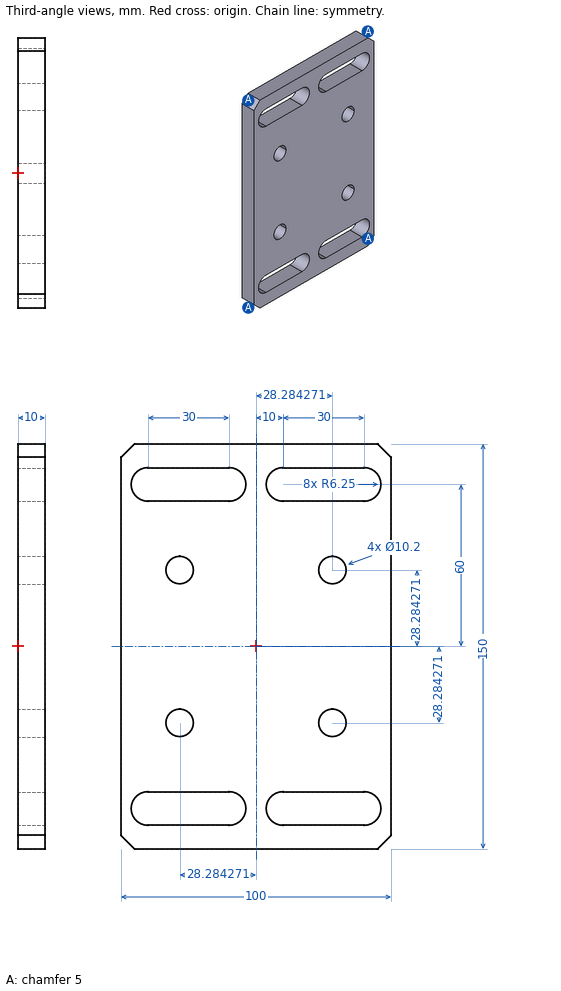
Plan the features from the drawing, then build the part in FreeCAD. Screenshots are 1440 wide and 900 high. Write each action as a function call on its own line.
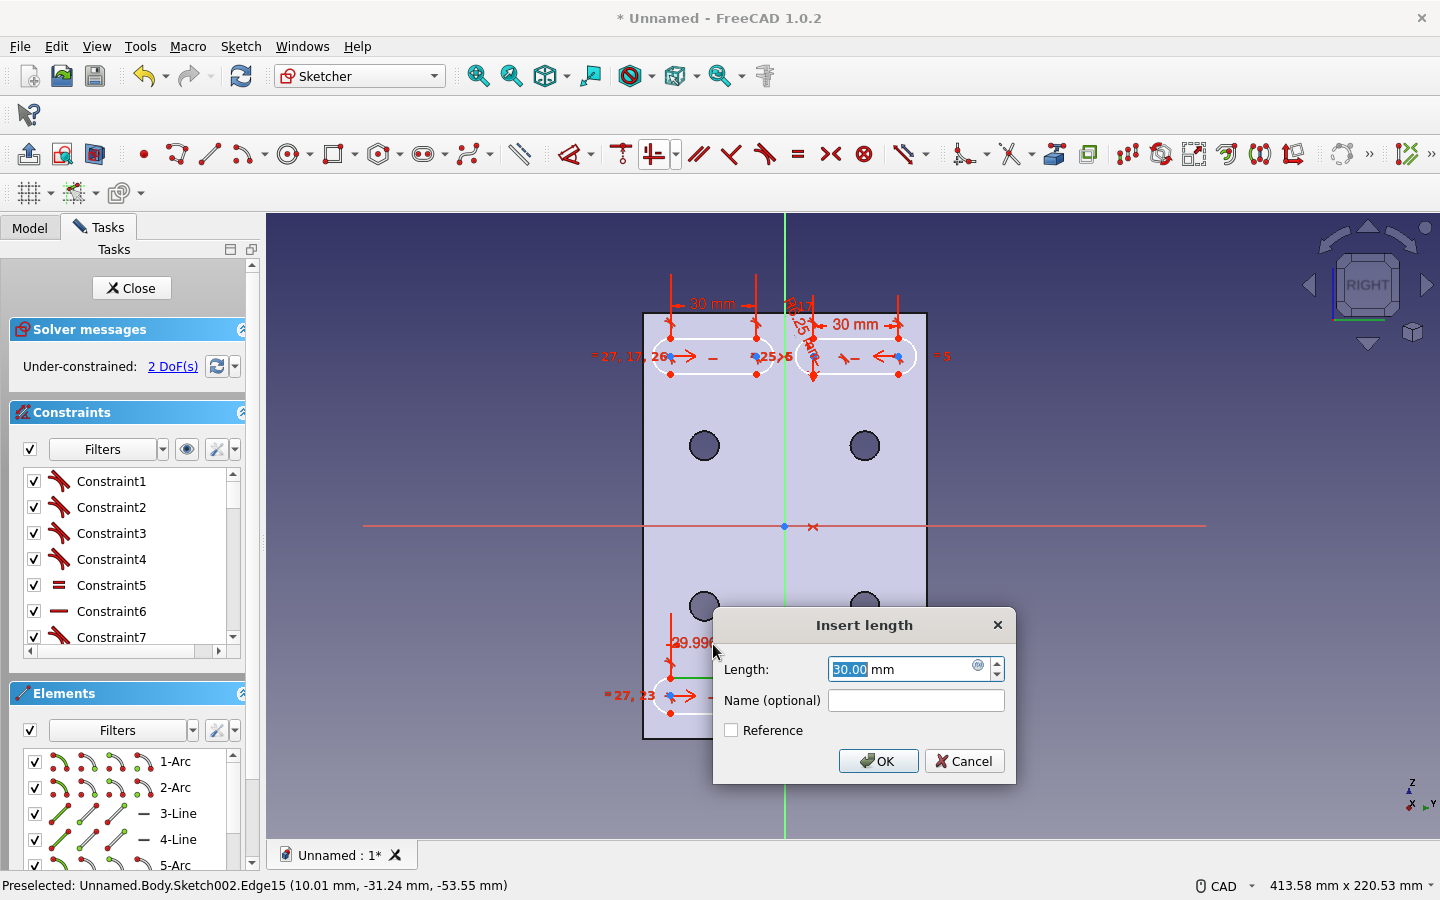
text(30)
key(Return)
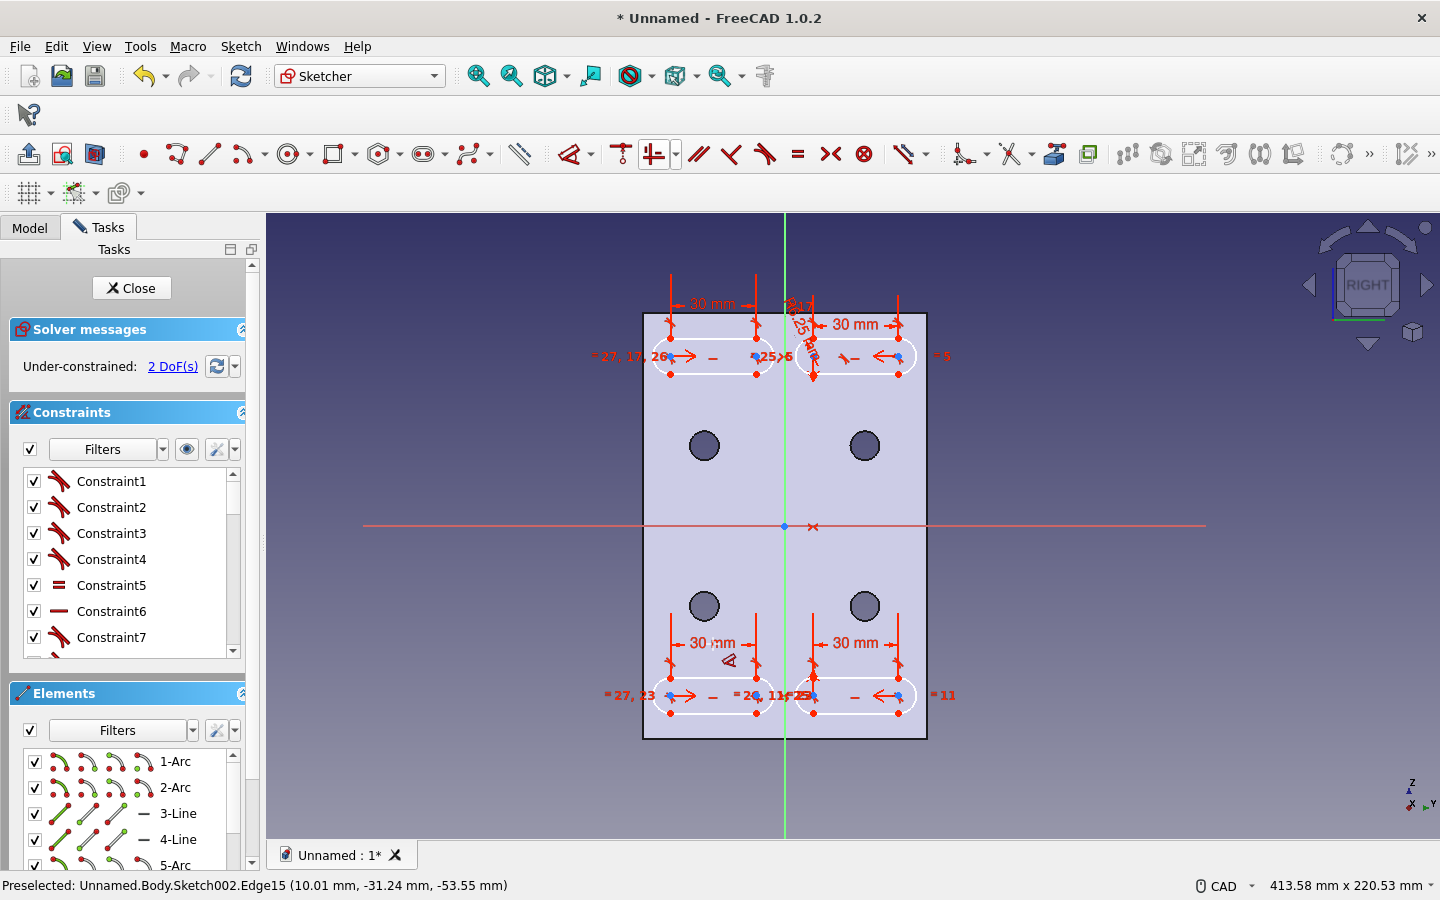
scroll(813, 339, up, 2)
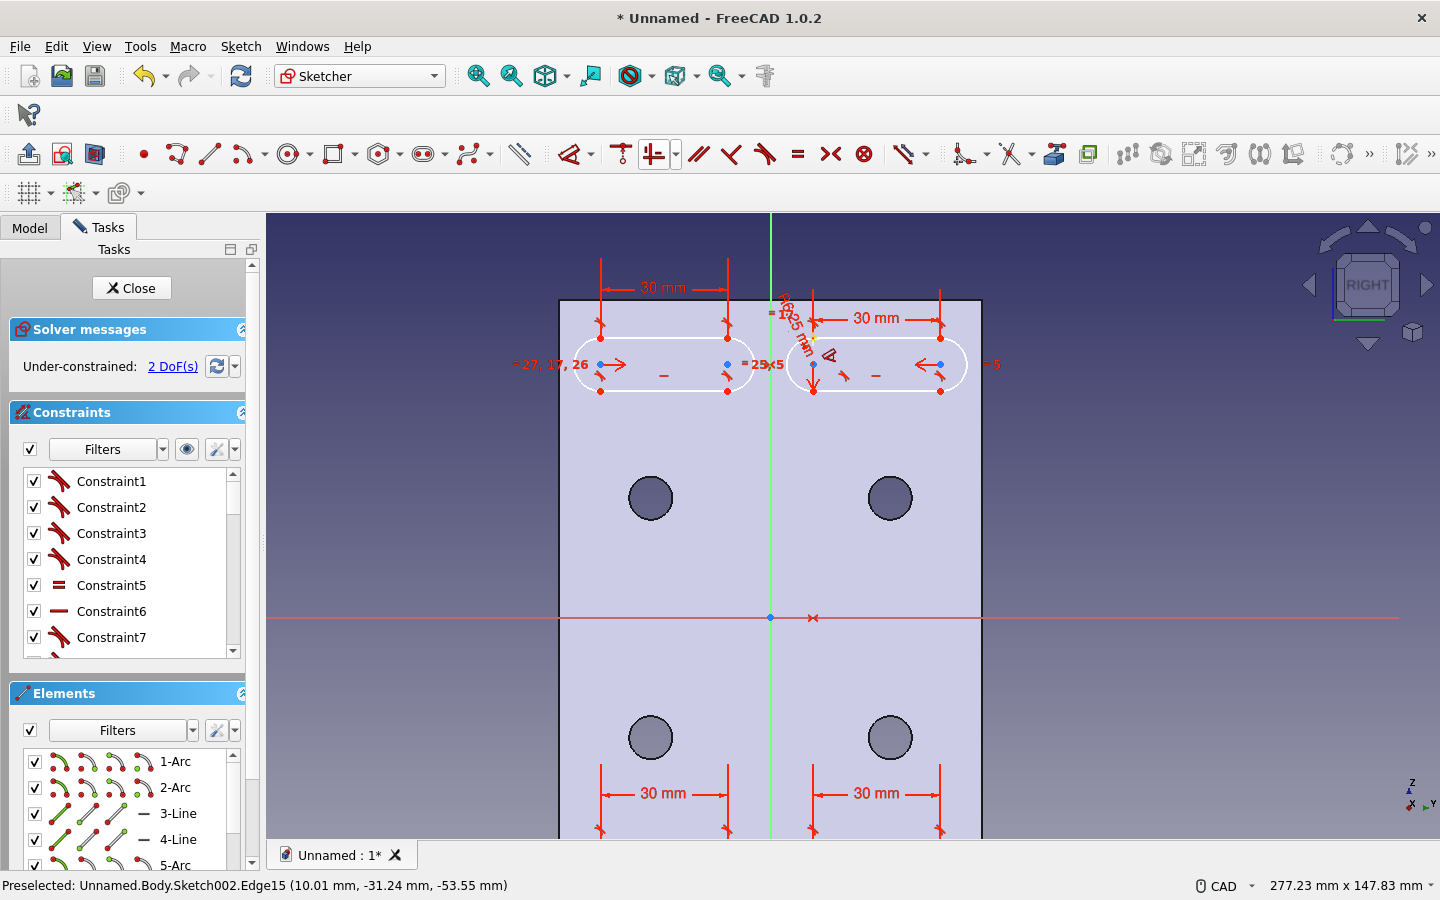
click(813, 338)
click(792, 304)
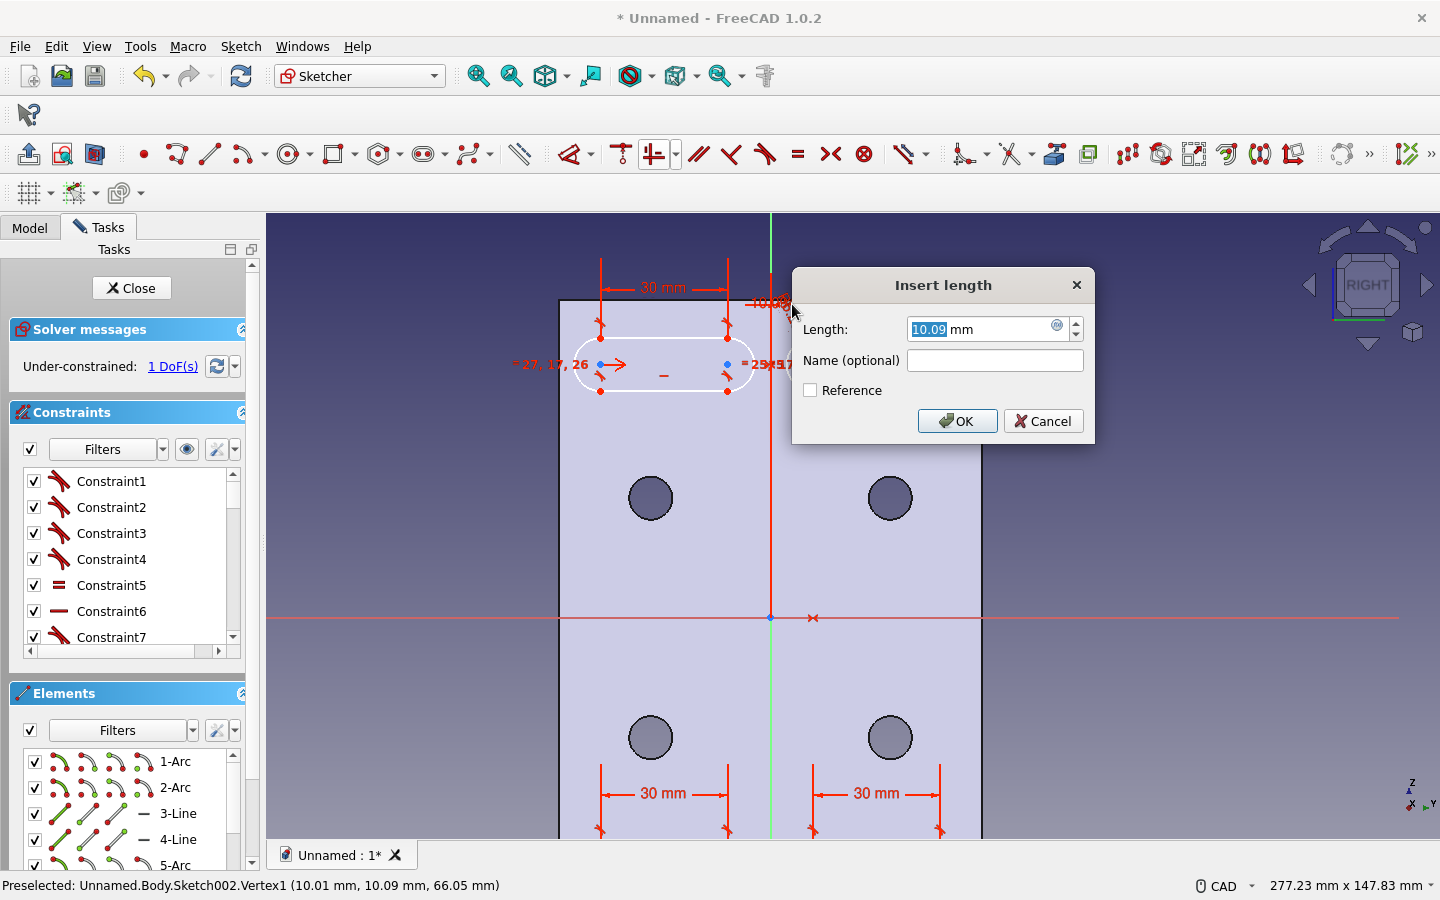
text(10)
key(Return)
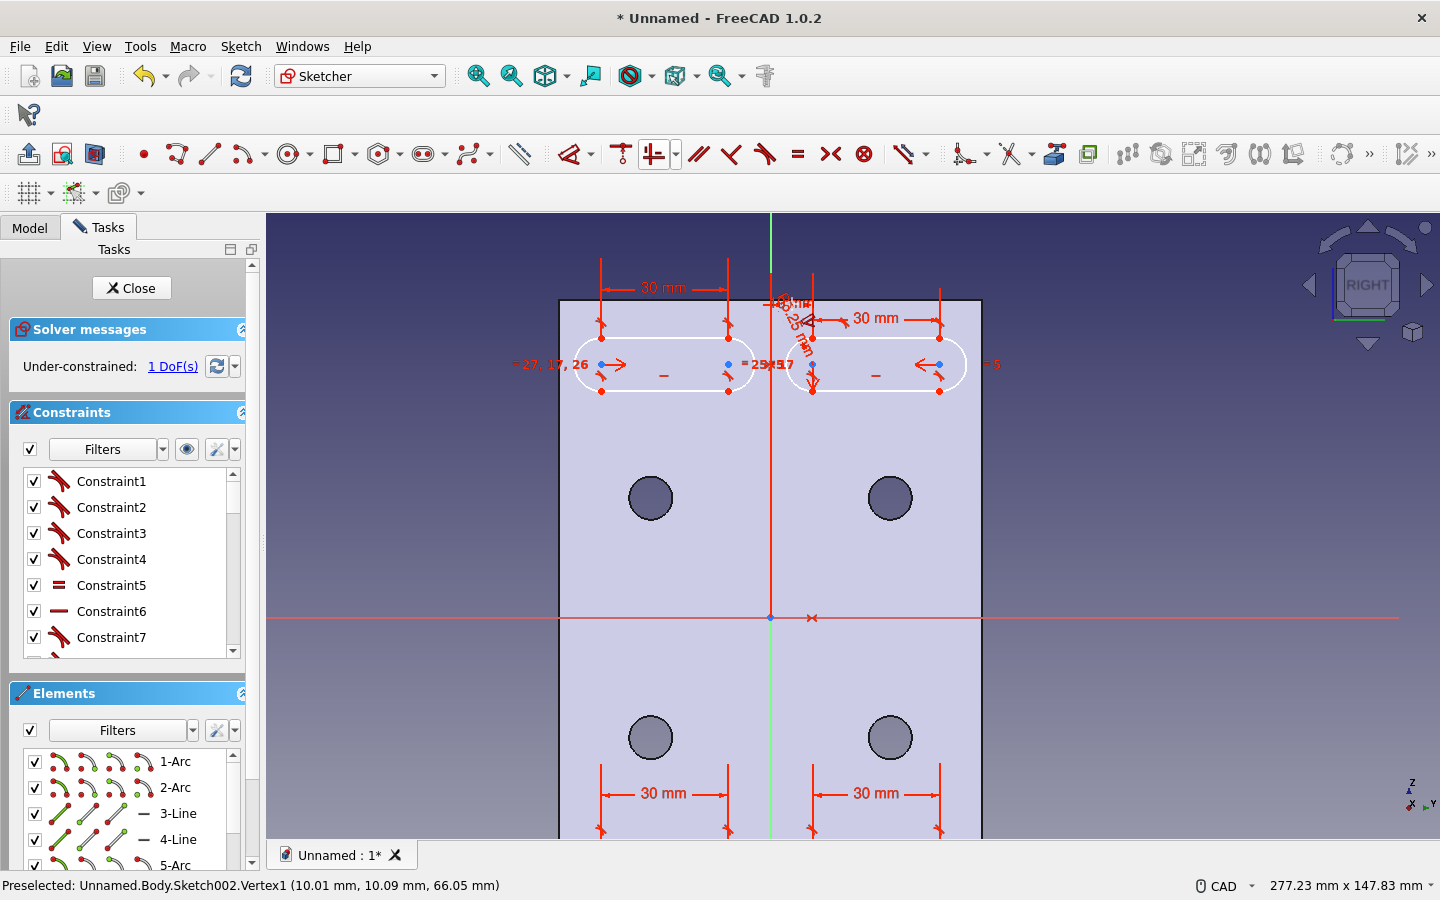
click(813, 365)
click(847, 491)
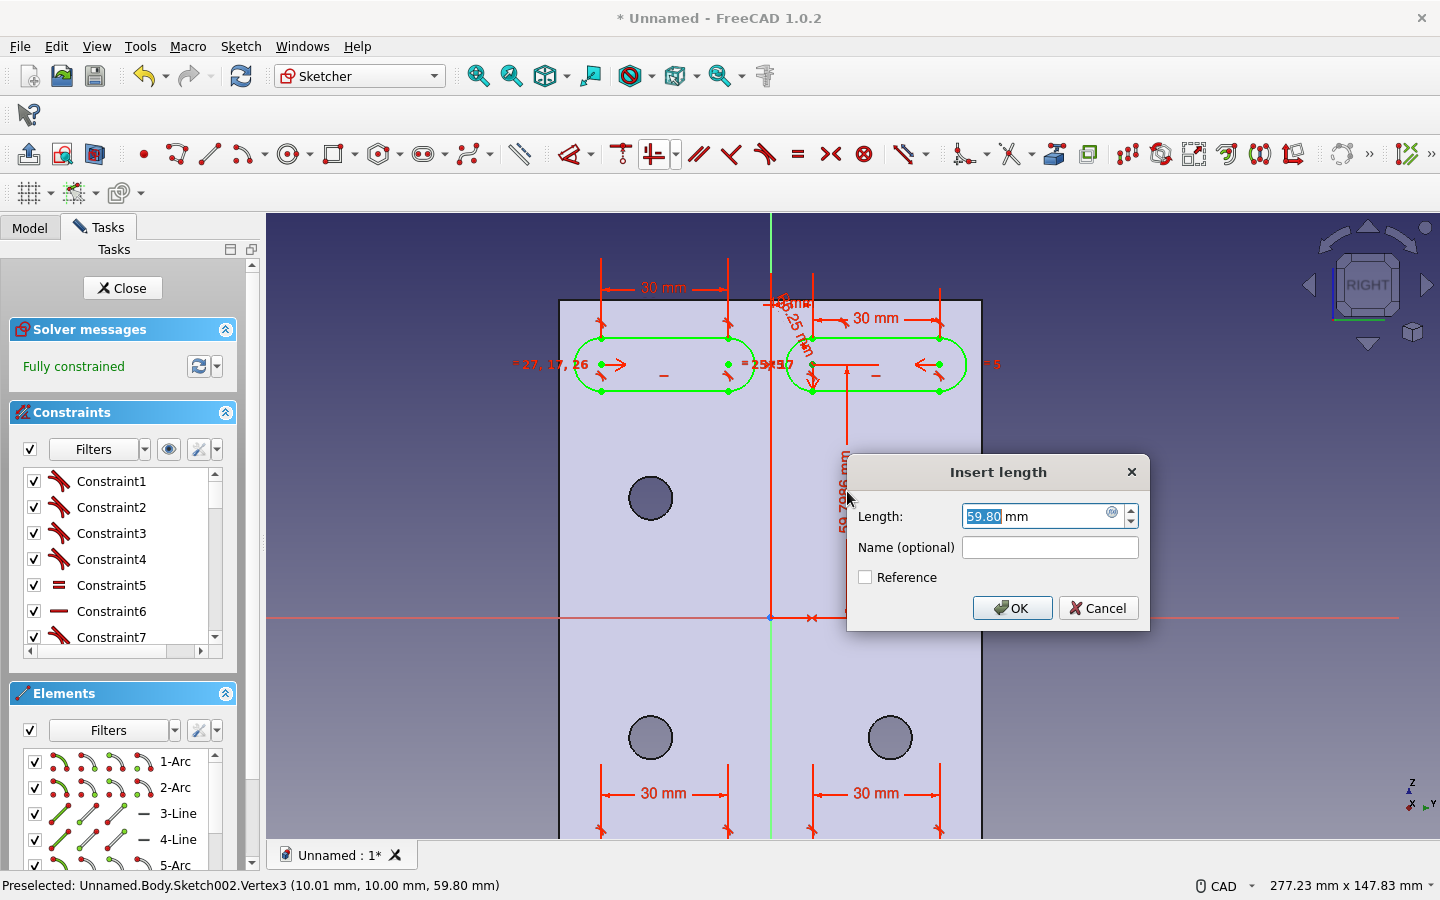
text(60)
key(Return)
key(Escape)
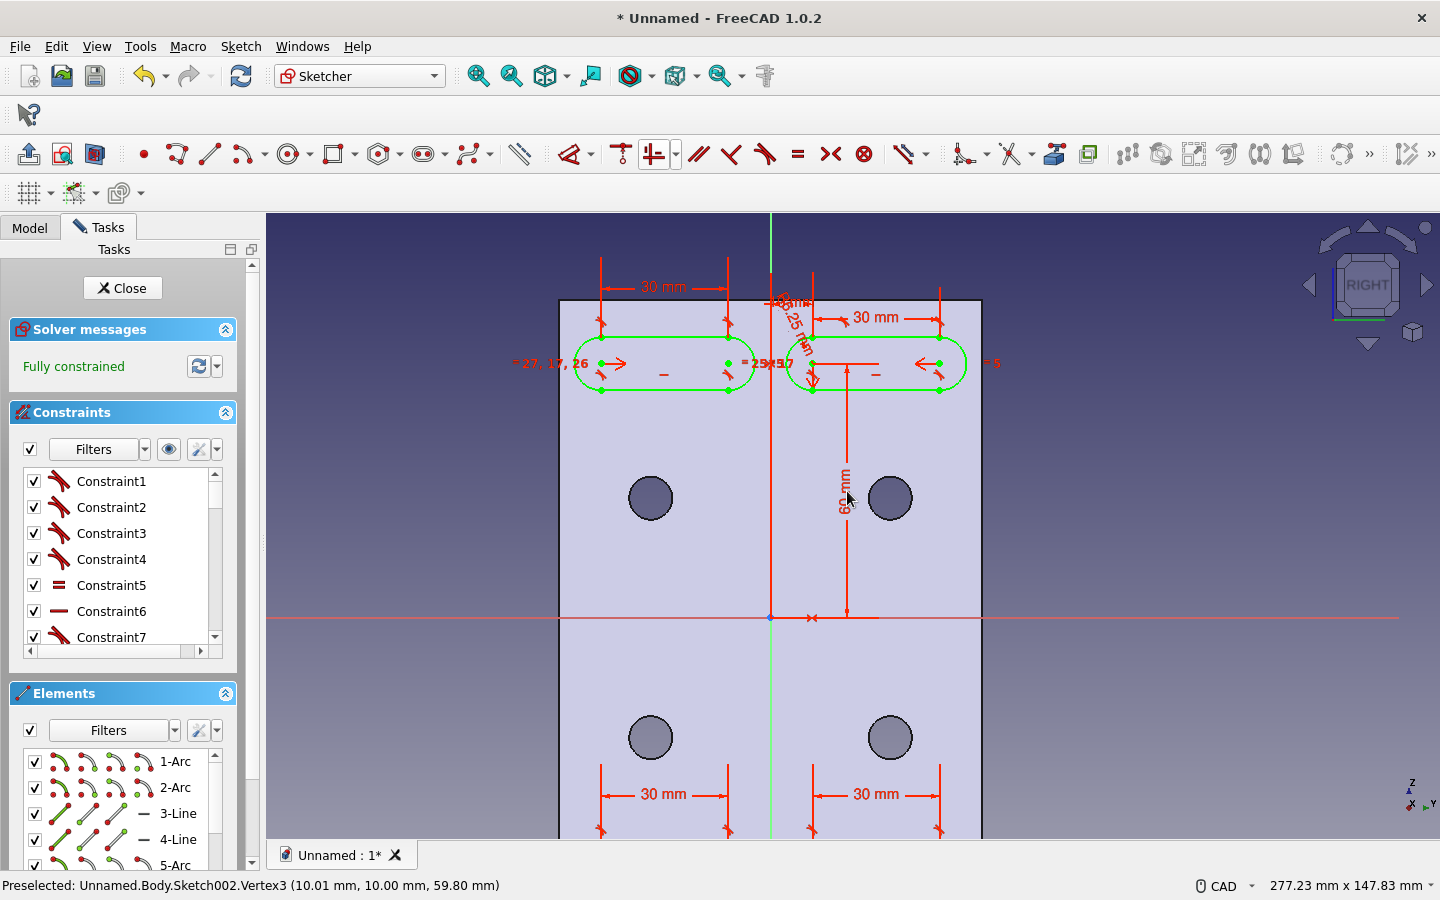
click(123, 288)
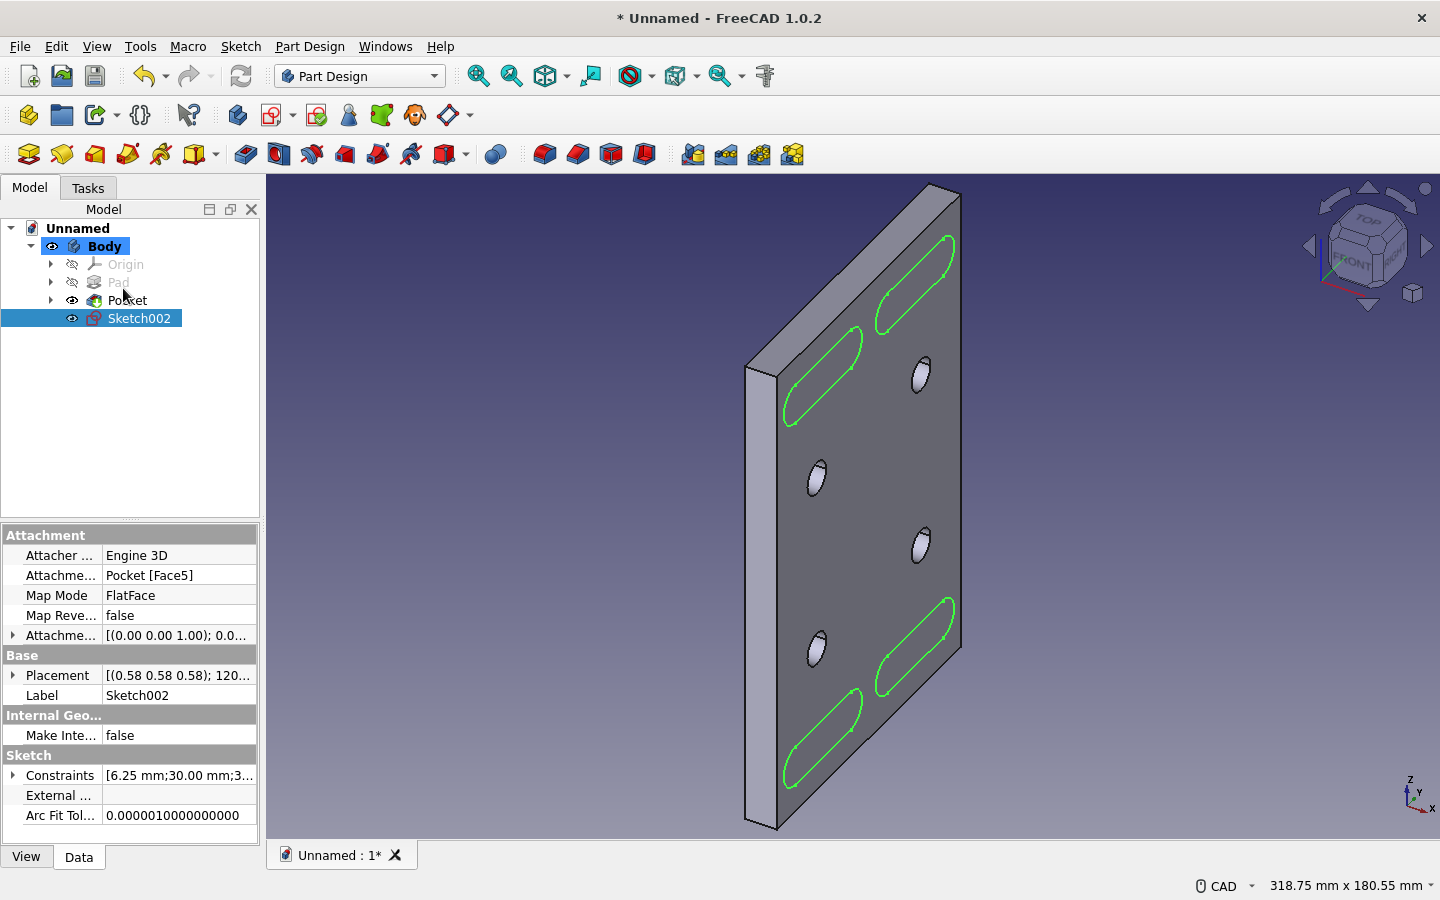
click(246, 154)